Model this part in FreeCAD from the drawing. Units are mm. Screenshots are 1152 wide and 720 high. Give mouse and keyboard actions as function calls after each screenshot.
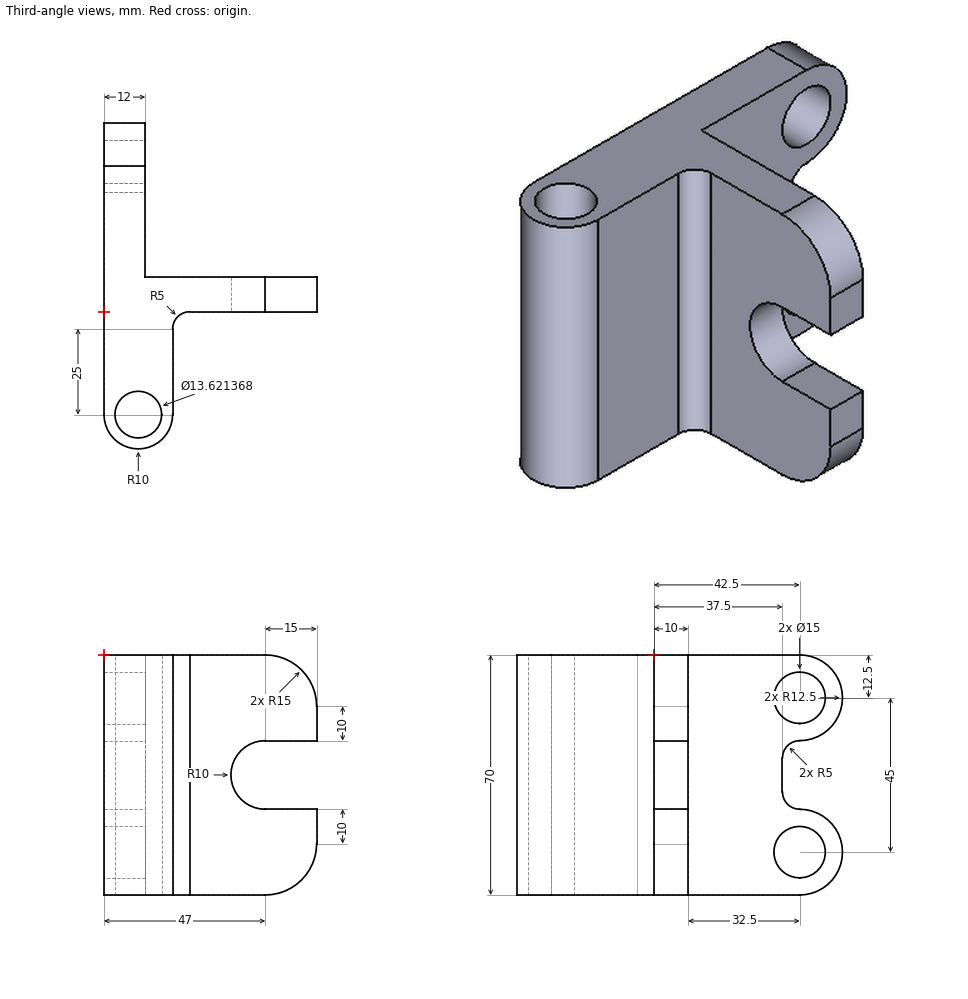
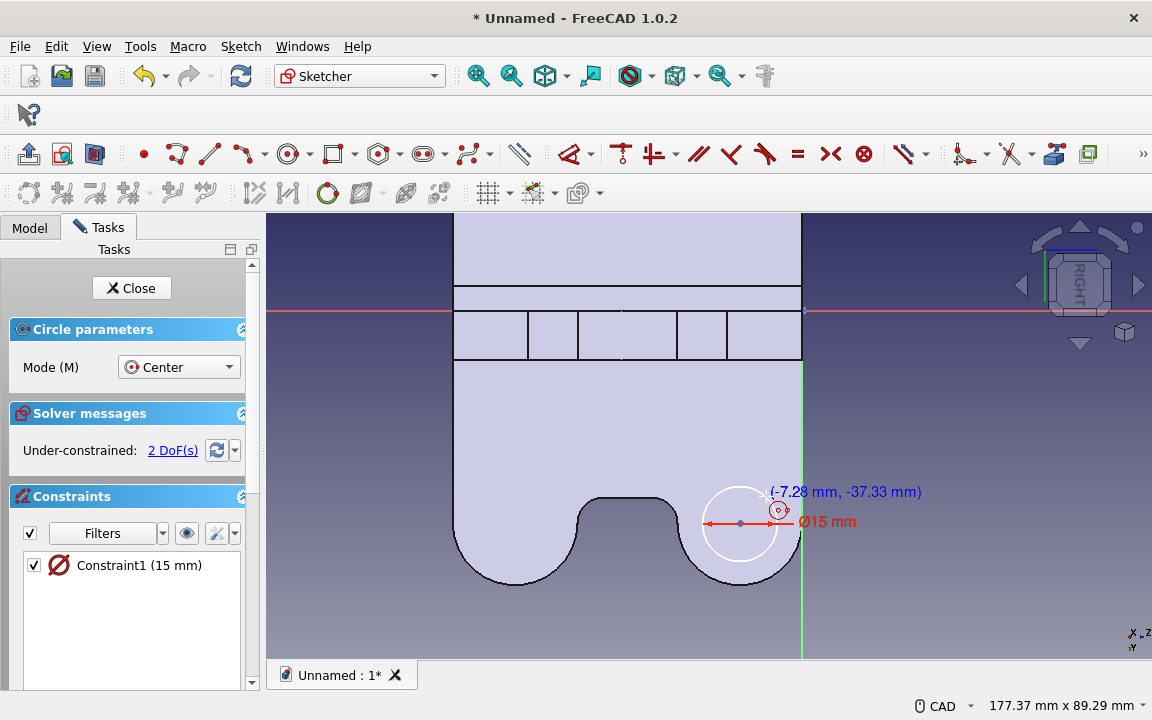
click(515, 523)
move(542, 496)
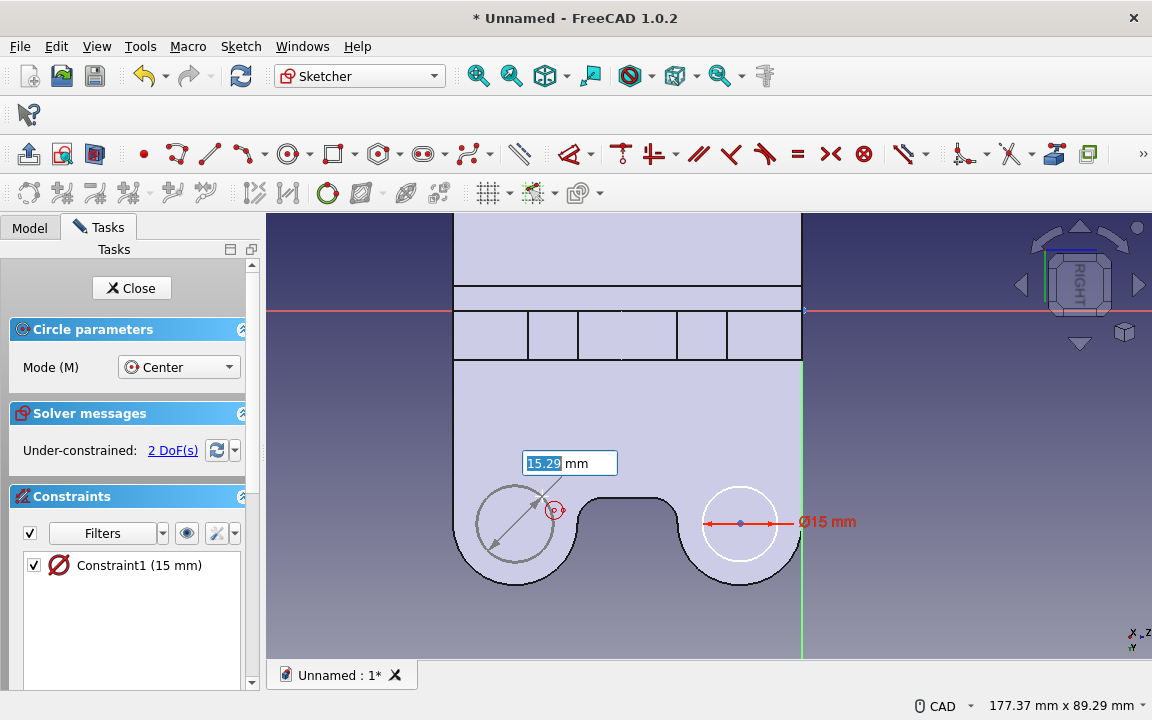
text(15)
key(Return)
key(Escape)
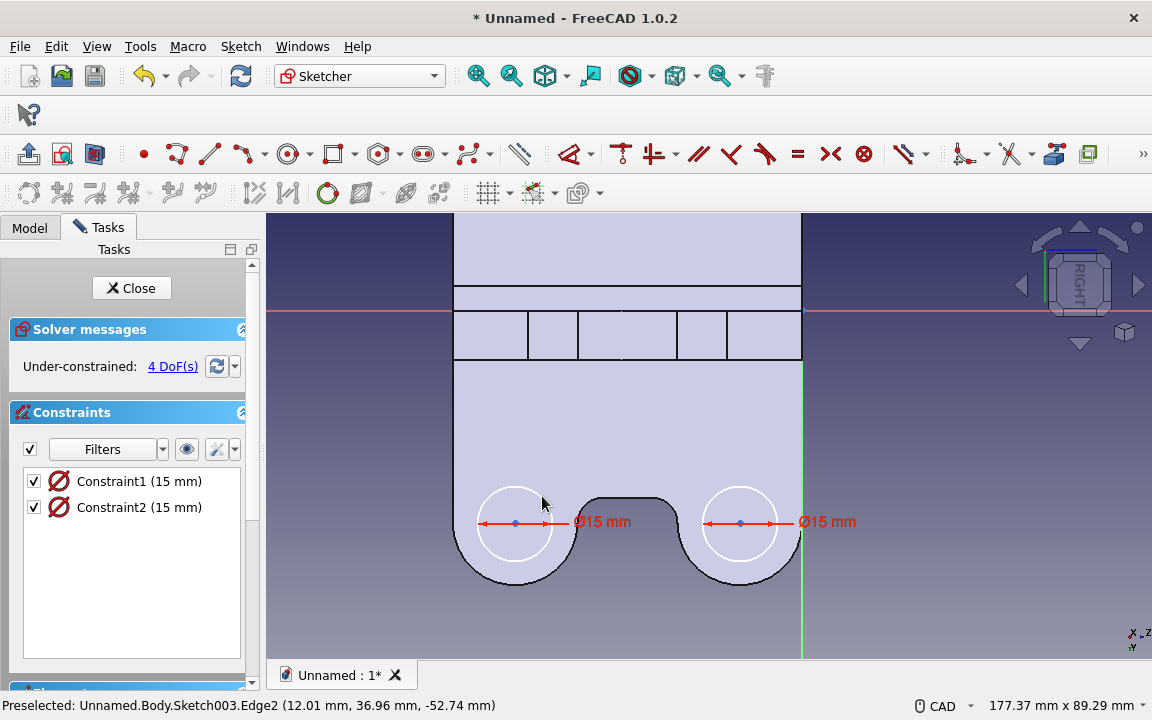
click(740, 524)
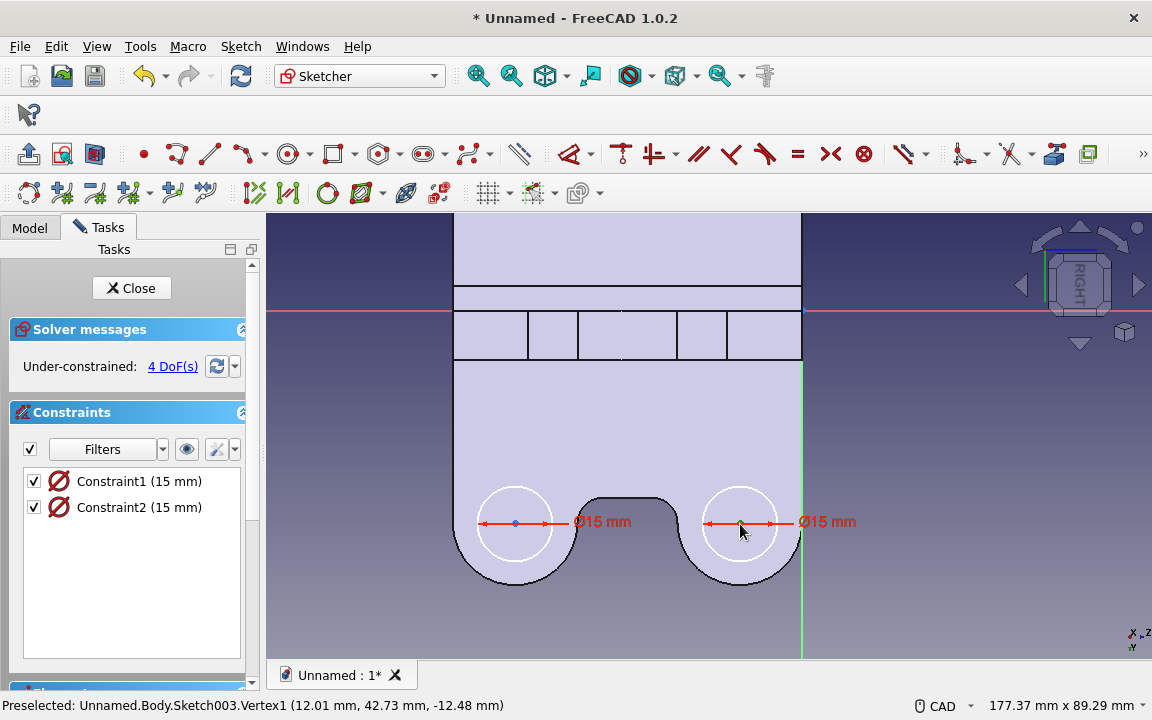
click(515, 524)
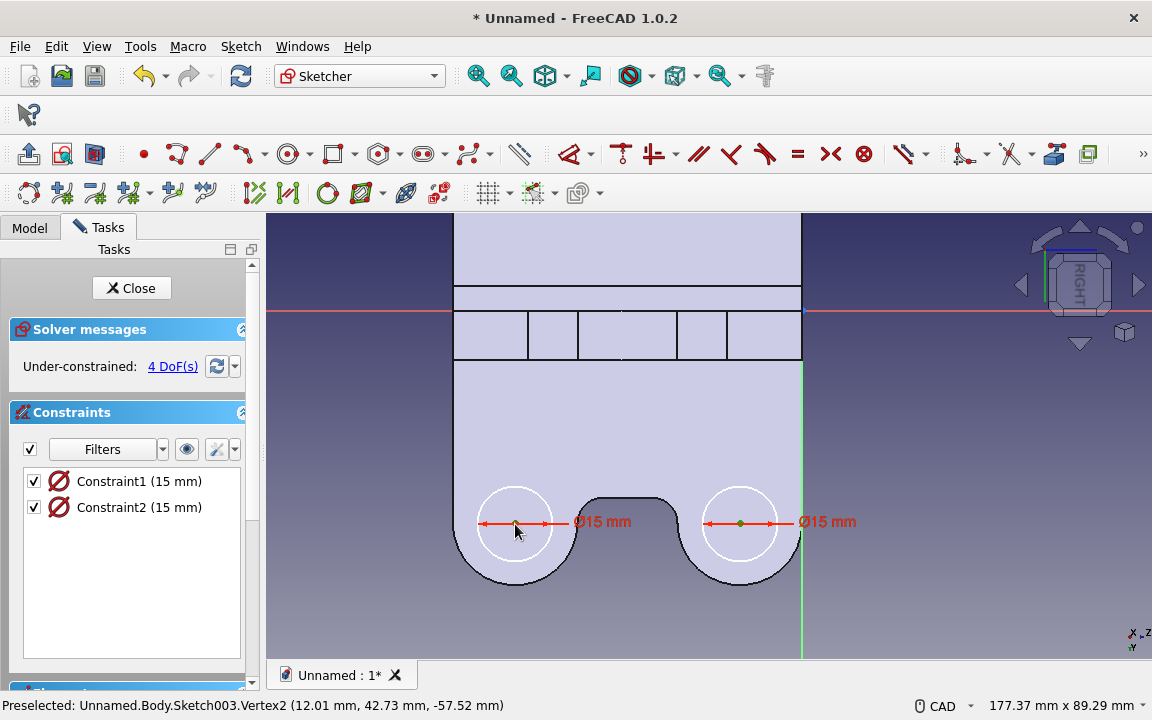
key(h)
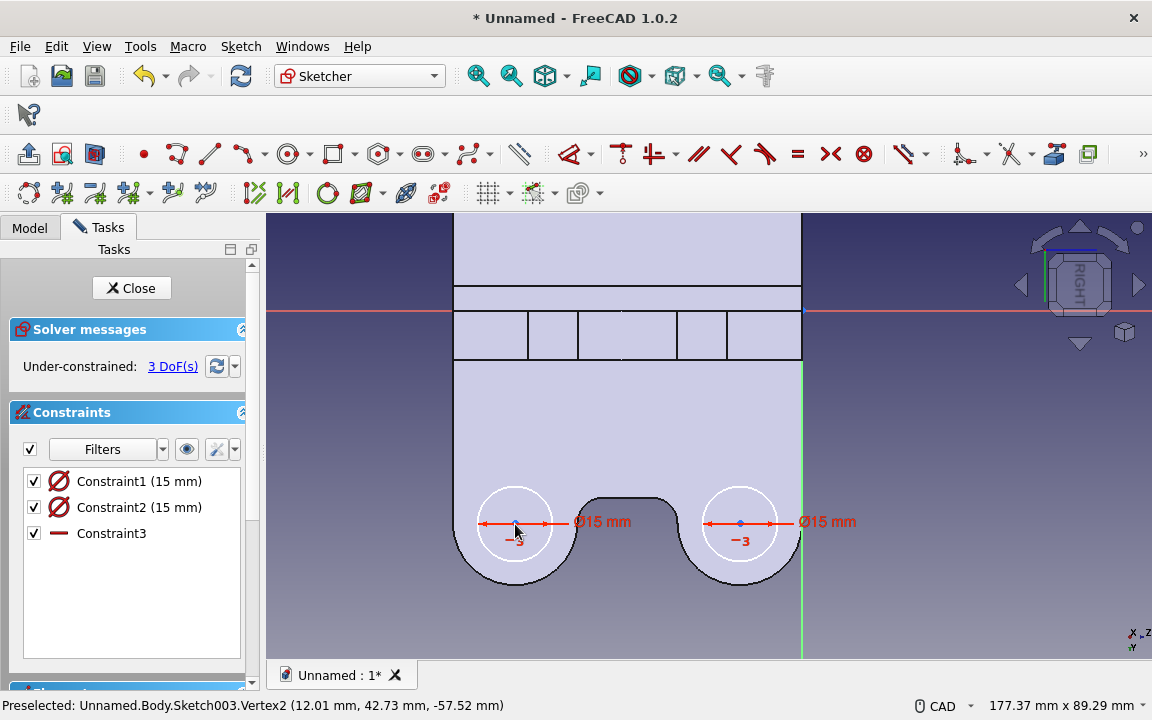
click(568, 154)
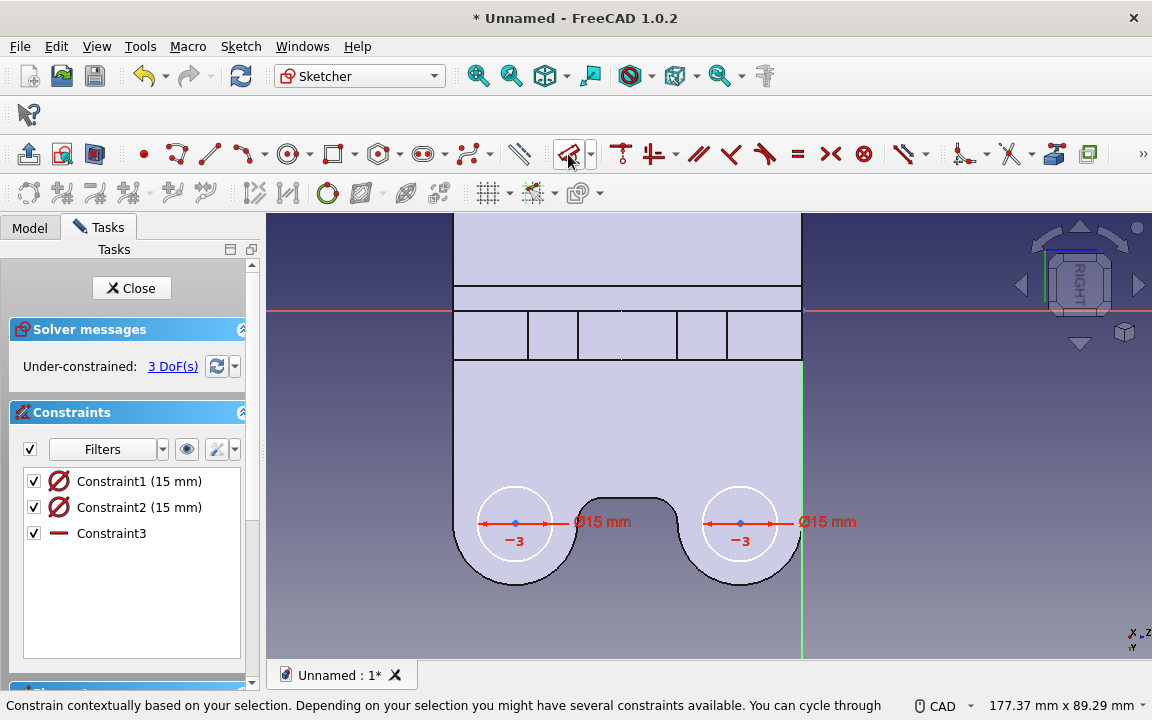
click(740, 524)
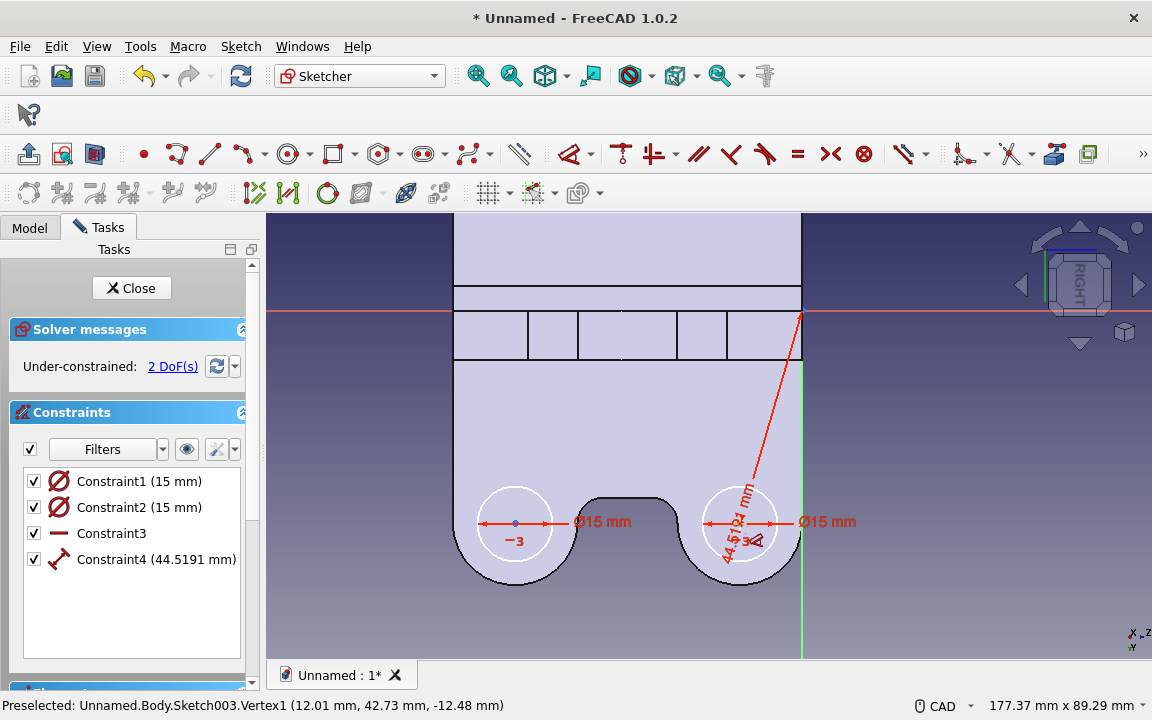
click(515, 524)
click(627, 558)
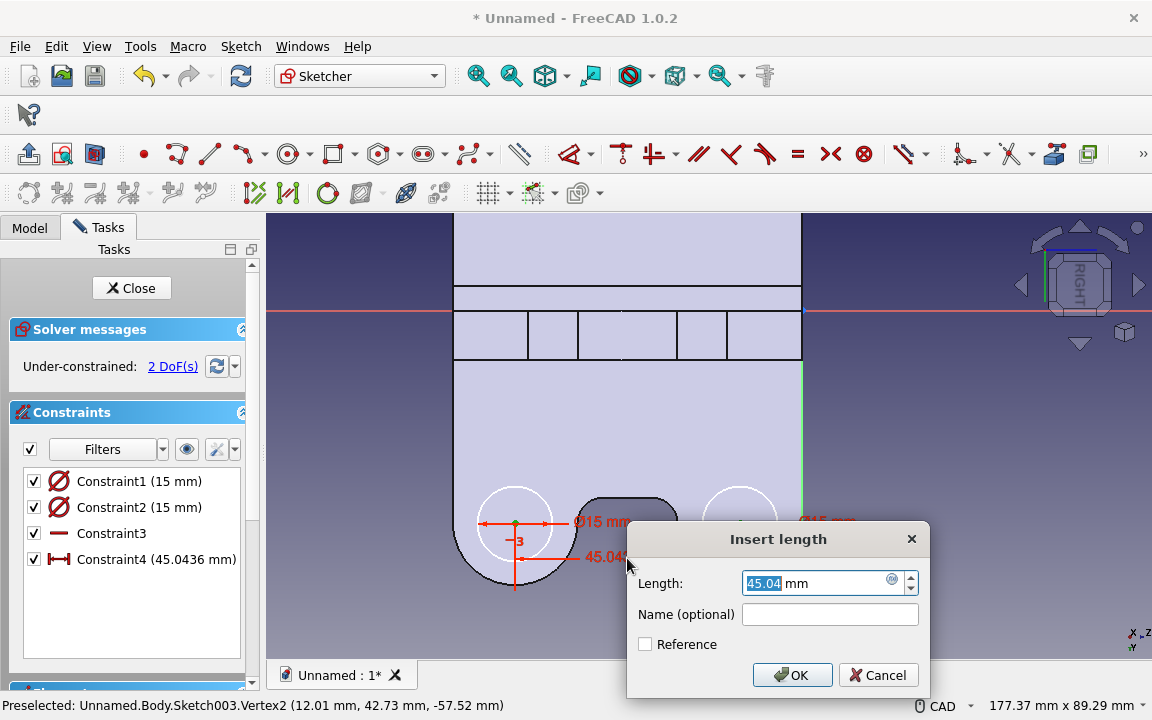
text(45)
key(Return)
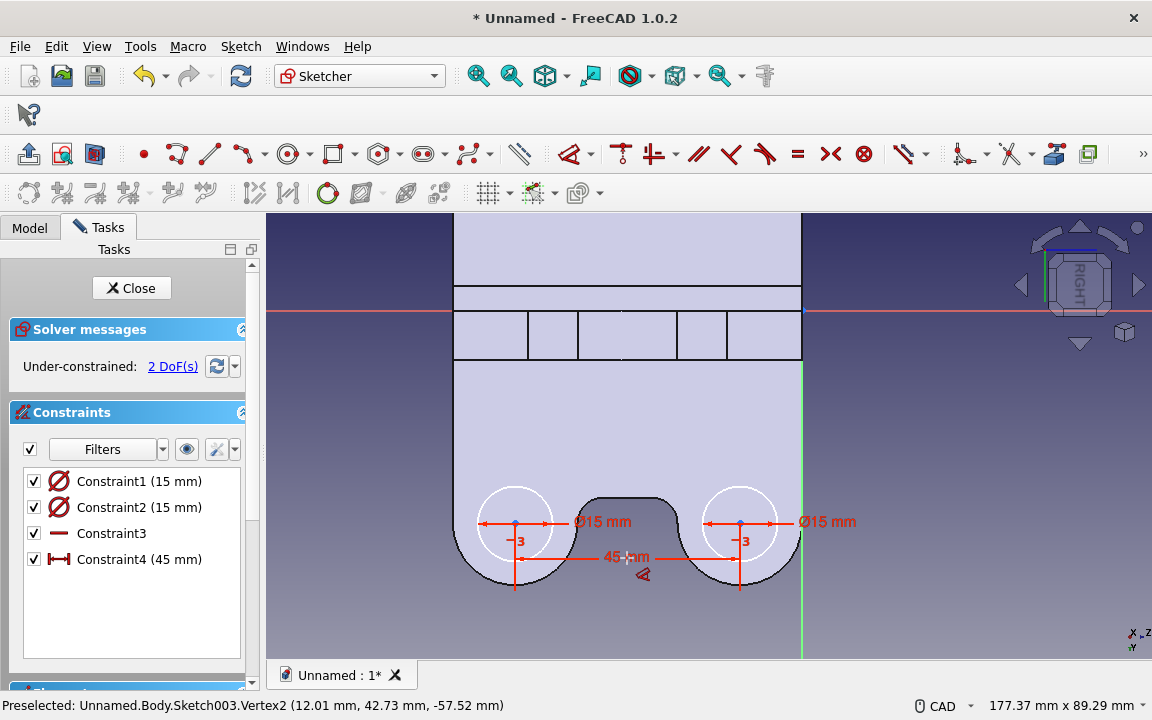
click(740, 524)
click(771, 277)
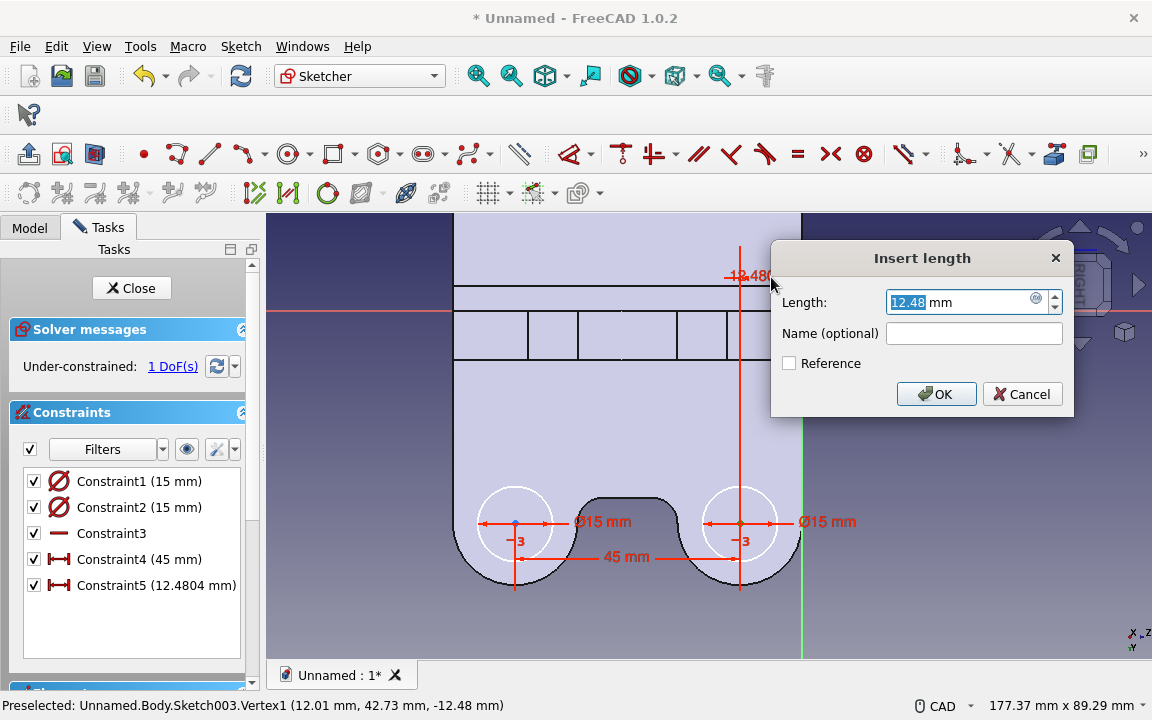
text(12.5)
key(Return)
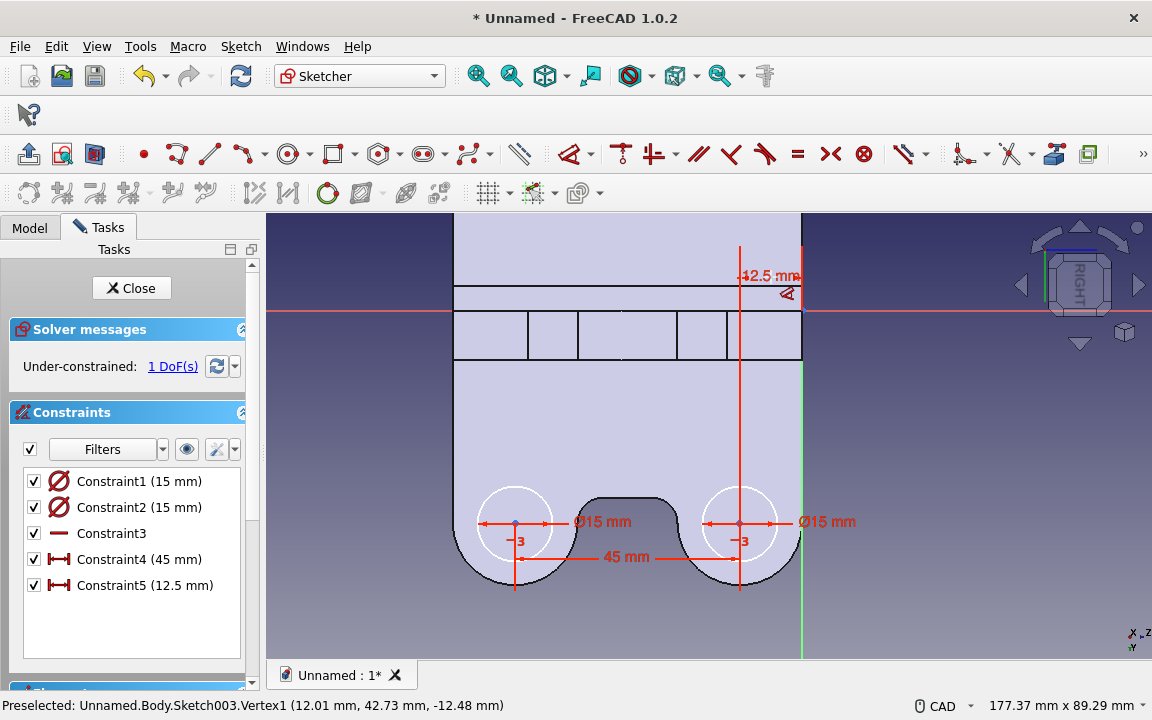
click(740, 524)
click(836, 417)